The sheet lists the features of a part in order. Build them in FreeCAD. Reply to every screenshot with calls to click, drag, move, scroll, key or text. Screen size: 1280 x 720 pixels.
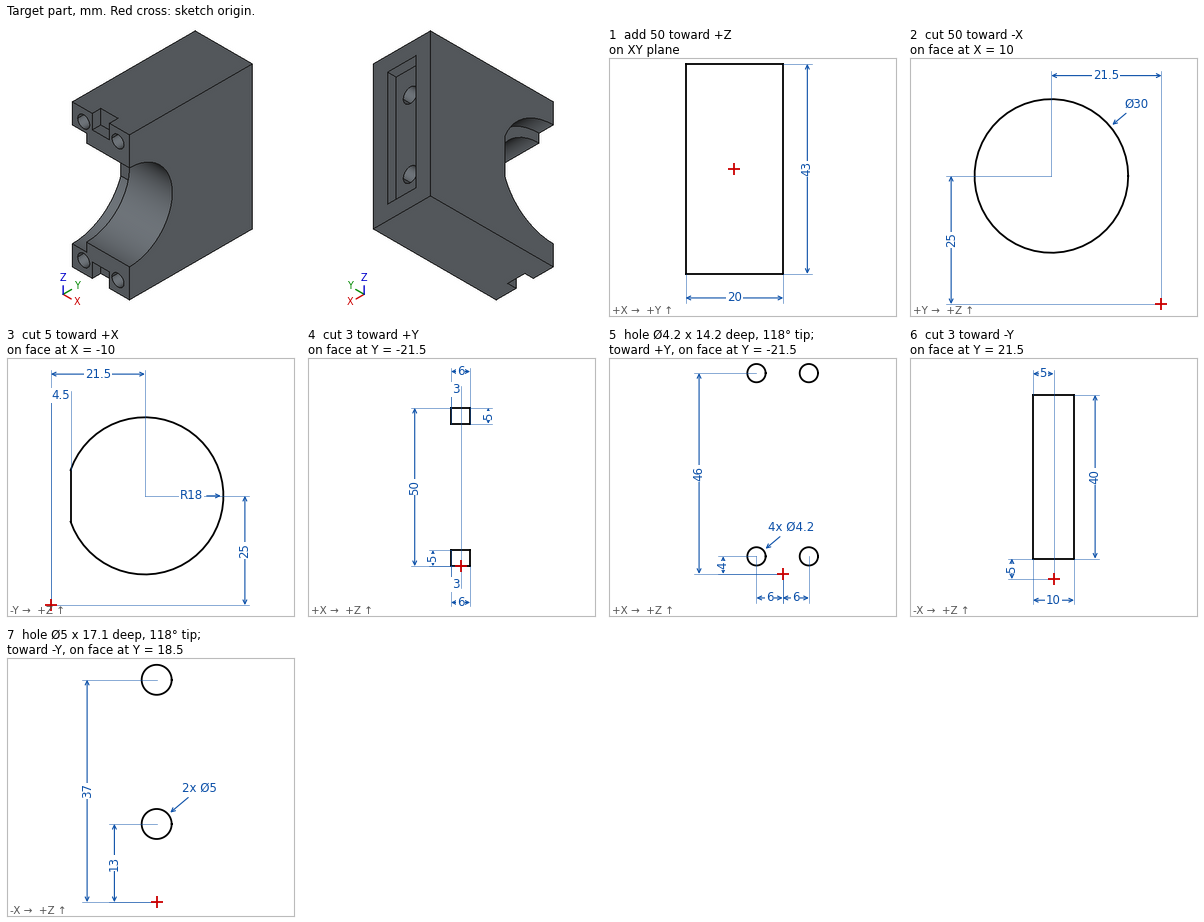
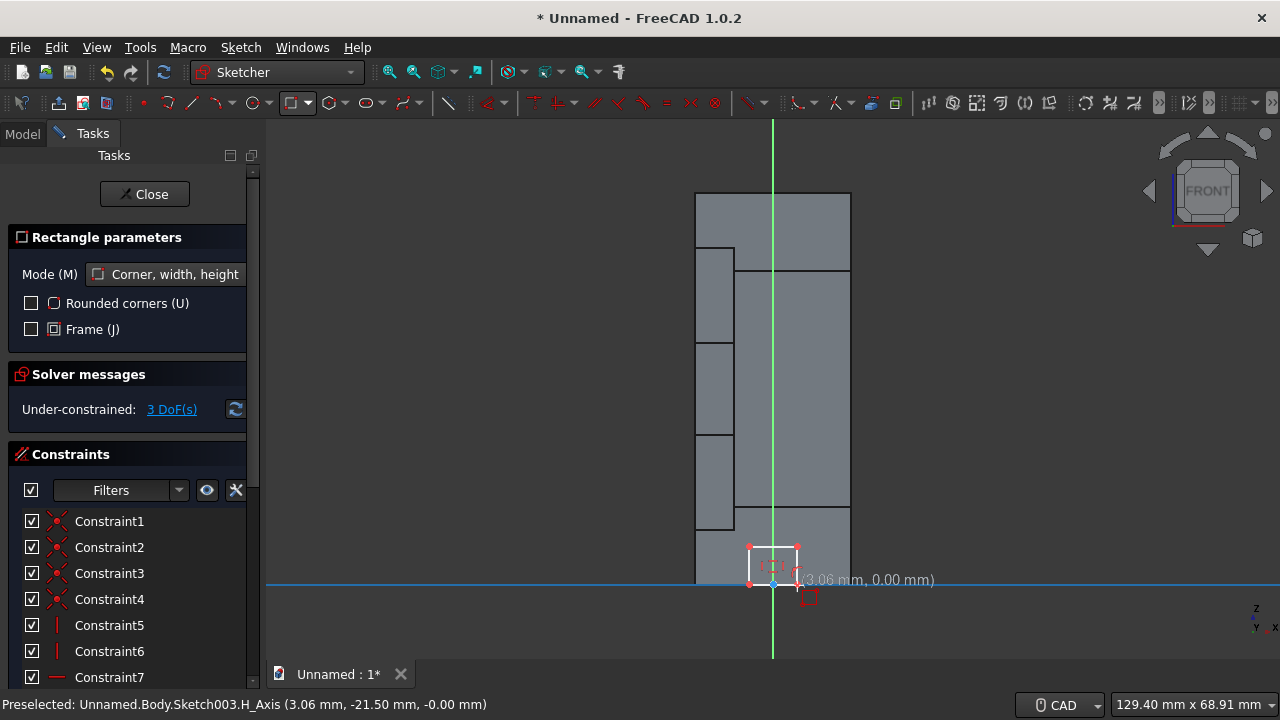
click(749, 193)
move(797, 232)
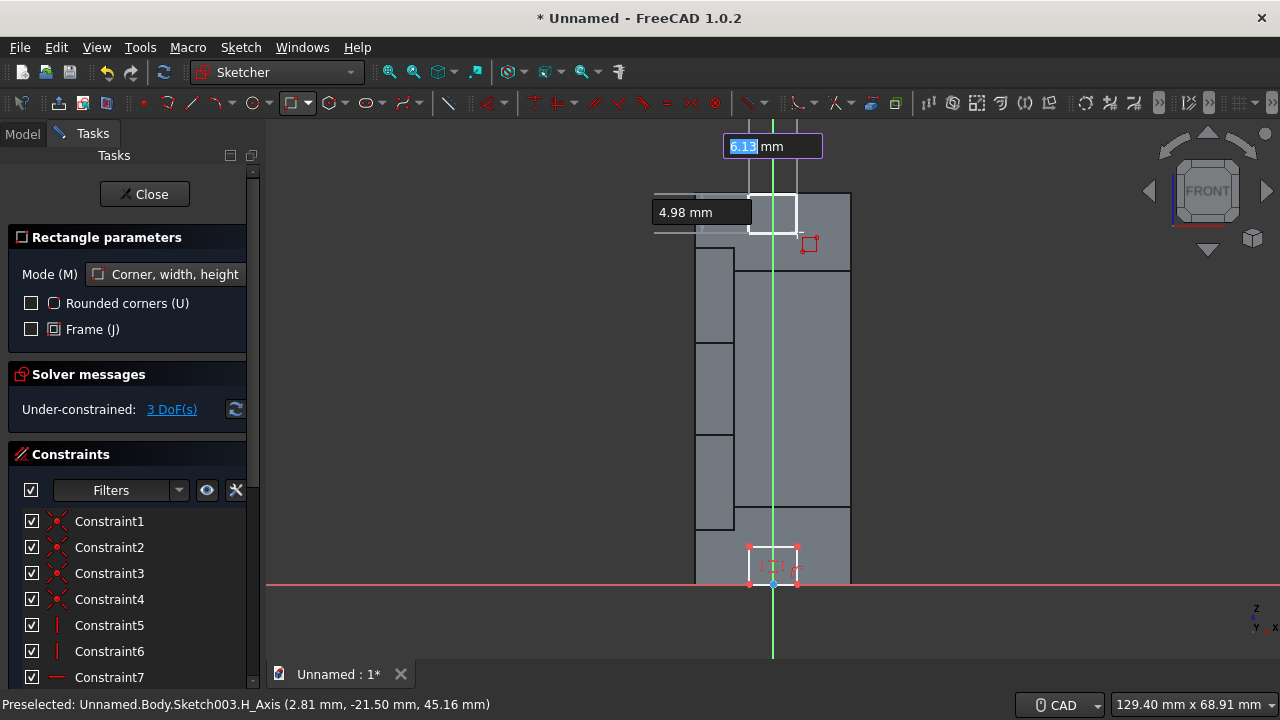
text(6)
key(Tab)
text(5)
key(Return)
key(Escape)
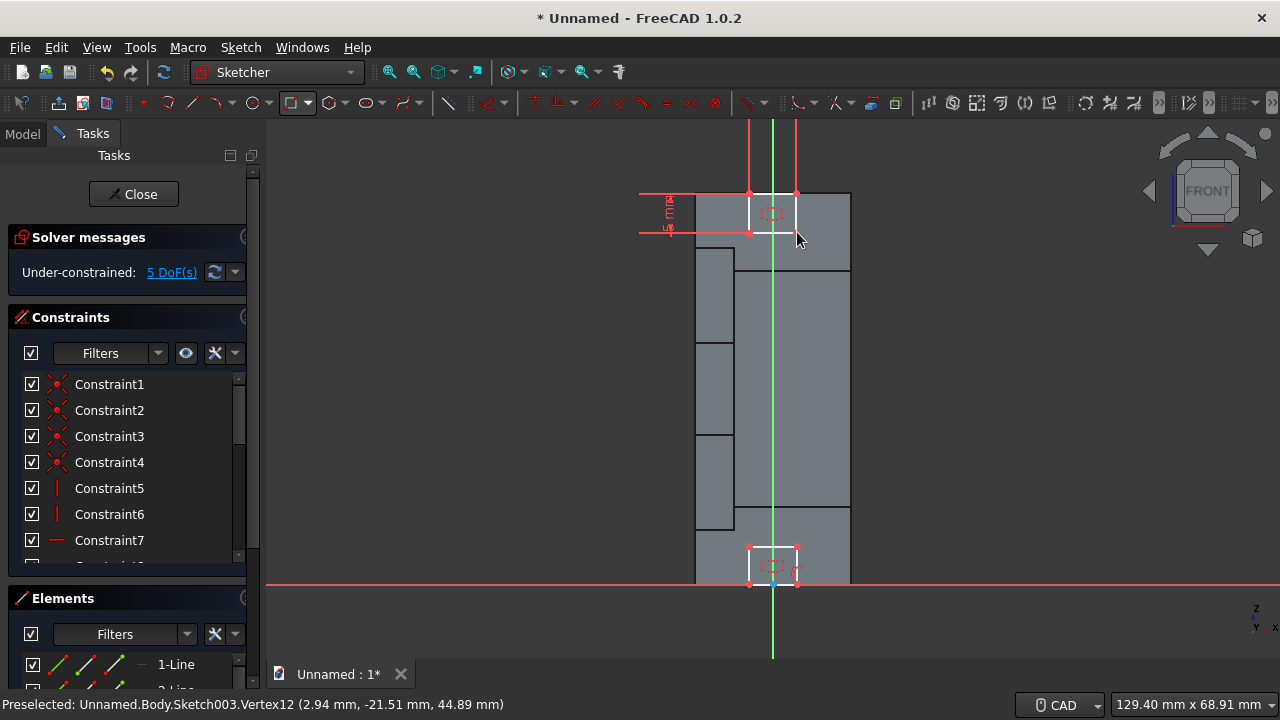
click(488, 104)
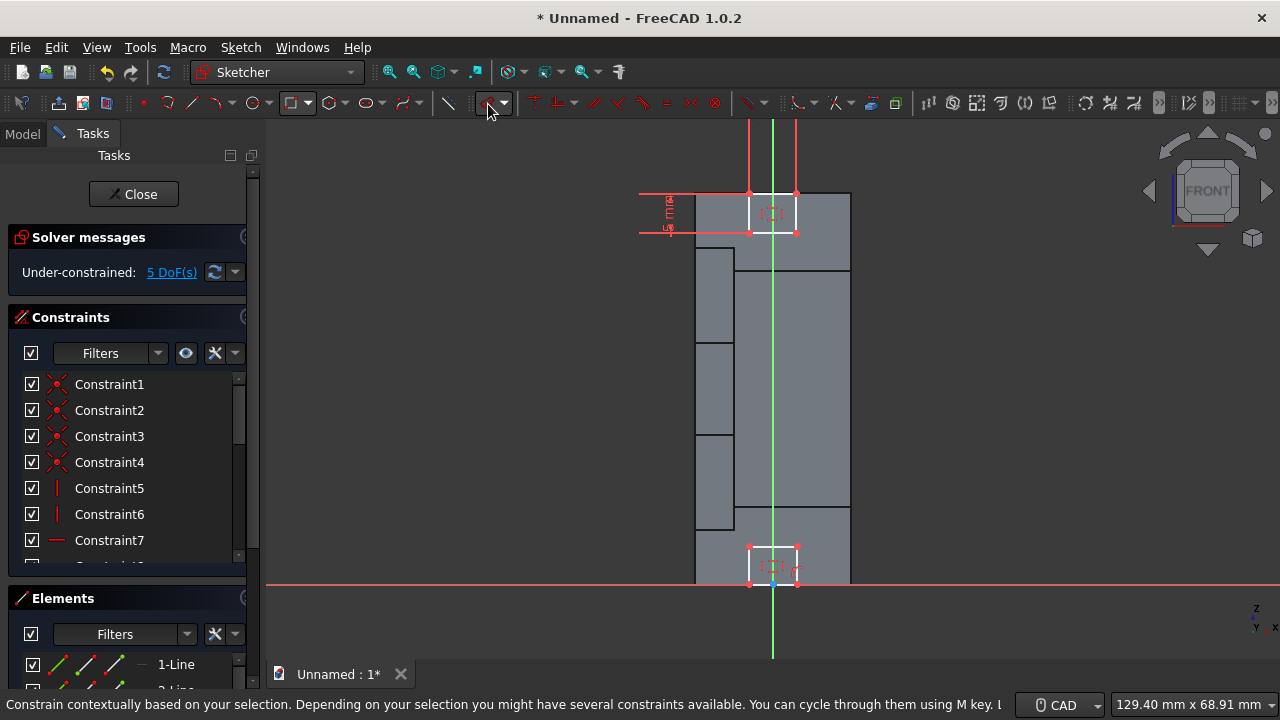
click(749, 558)
click(715, 566)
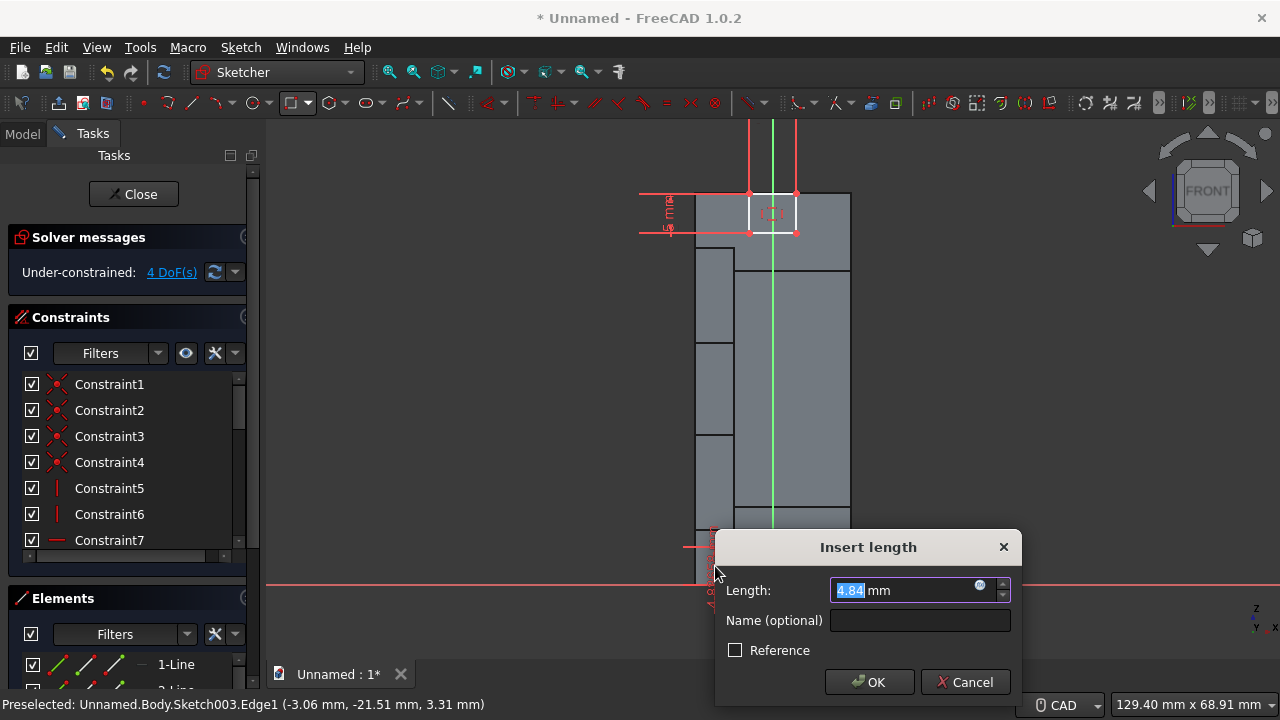
text(5)
key(Return)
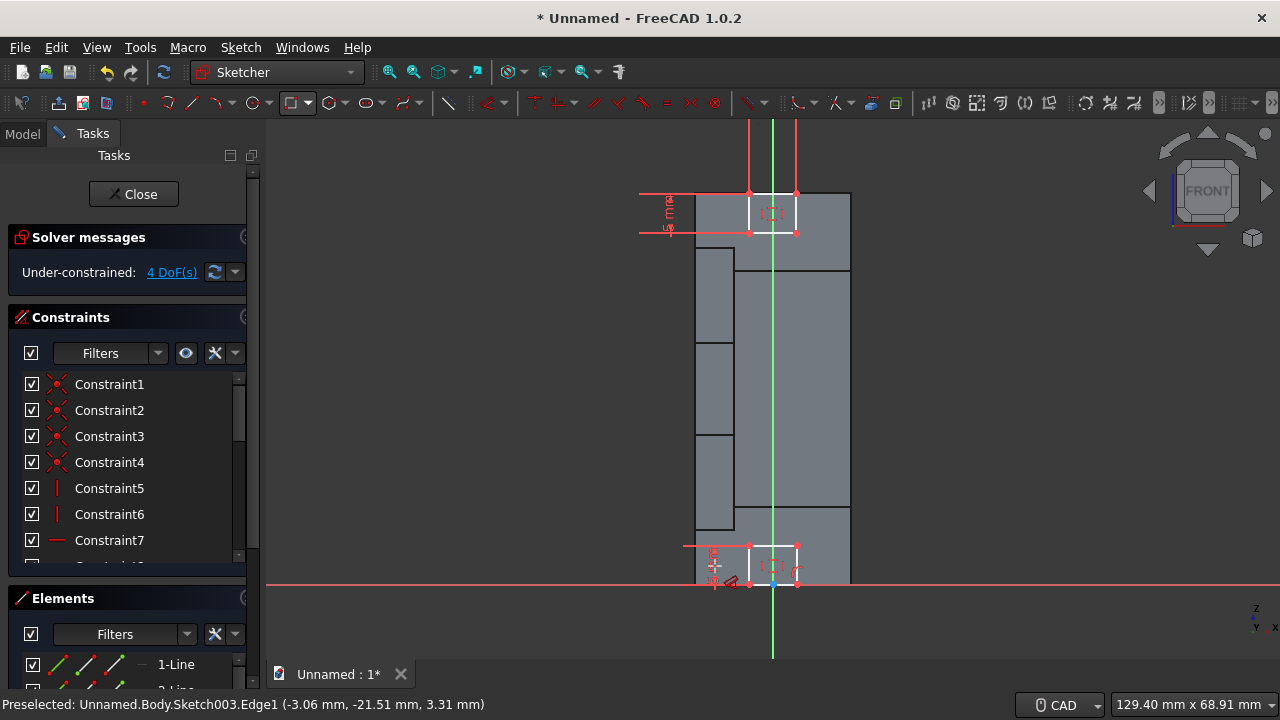
scroll(763, 585, up, 2)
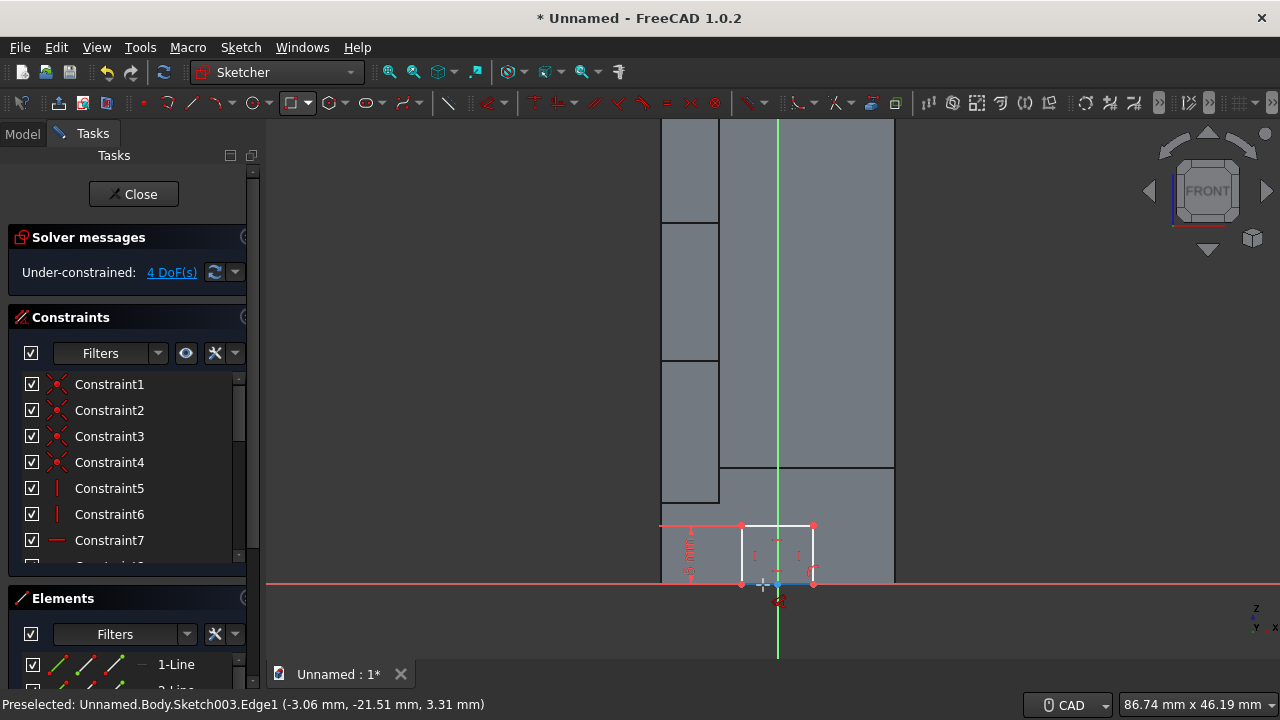
click(763, 584)
click(761, 618)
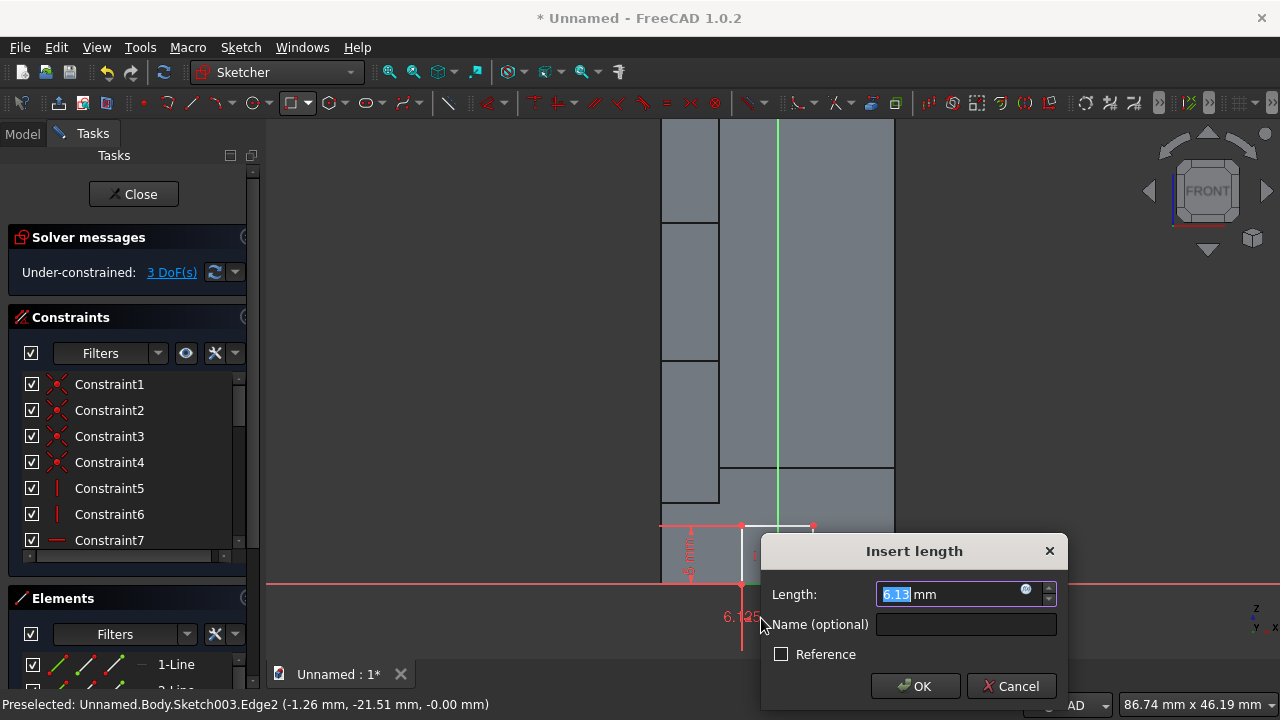
text(6)
key(Return)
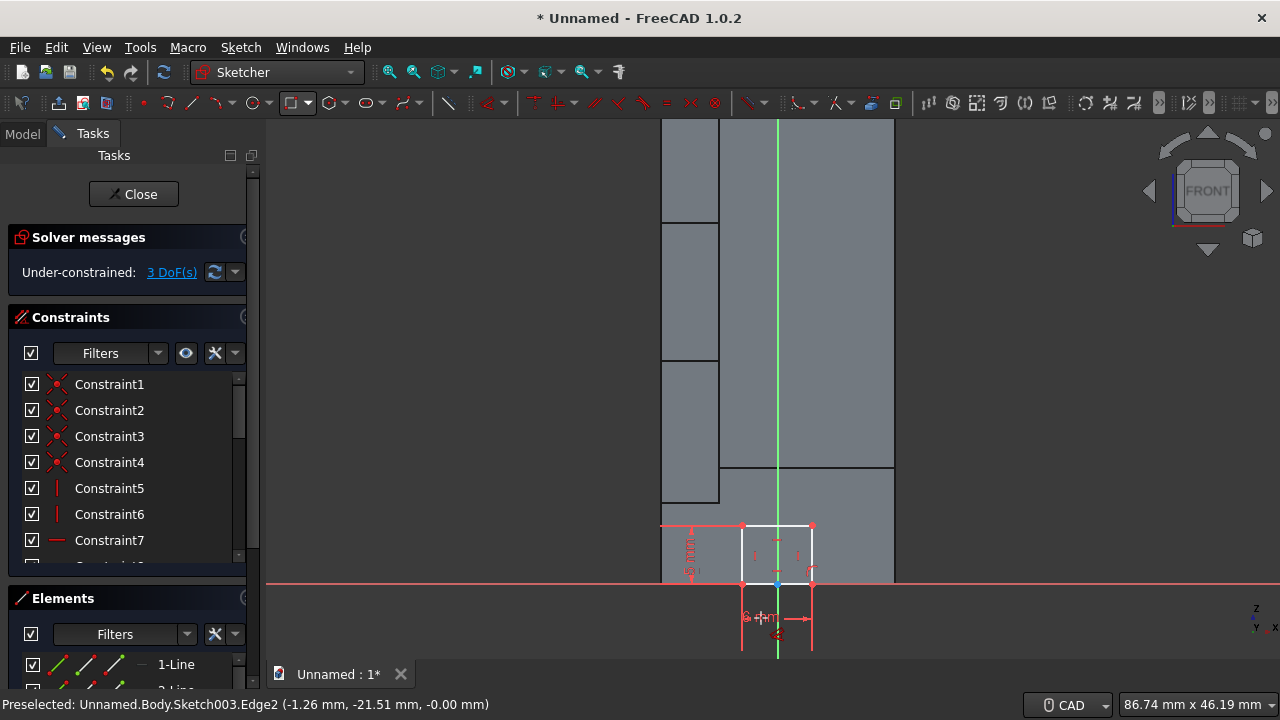
click(742, 526)
click(760, 492)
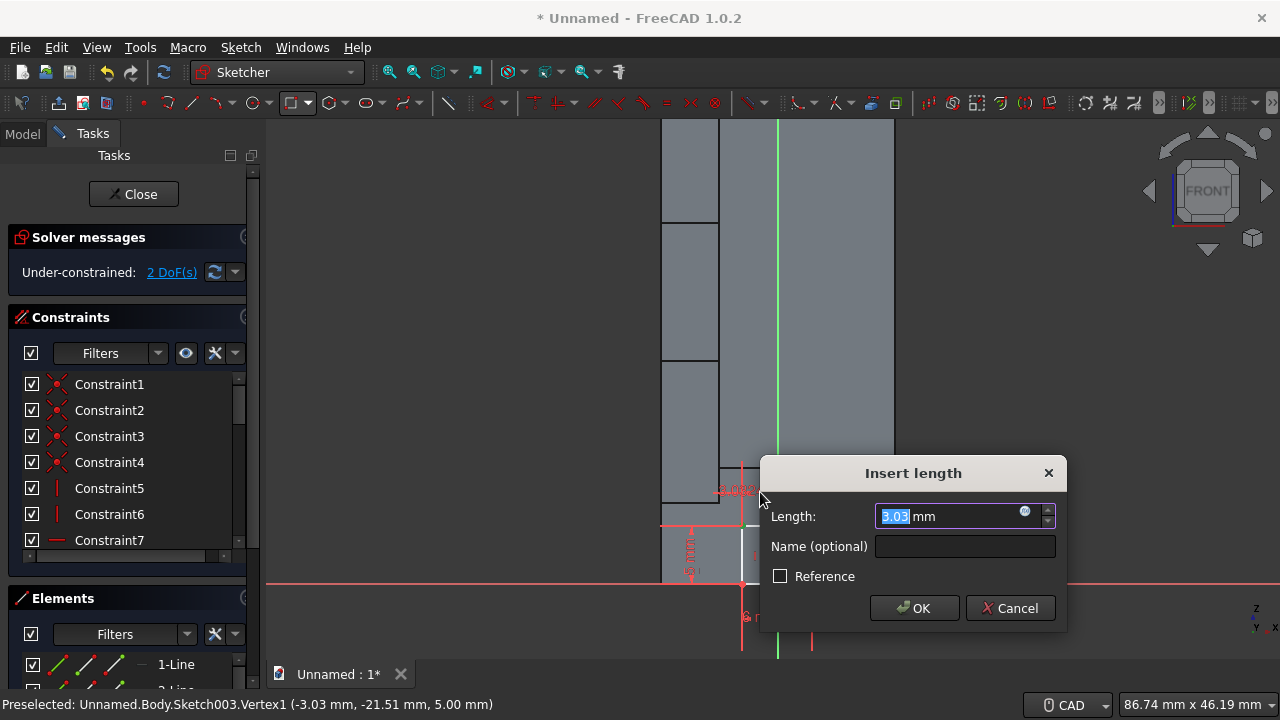
text(3)
key(Return)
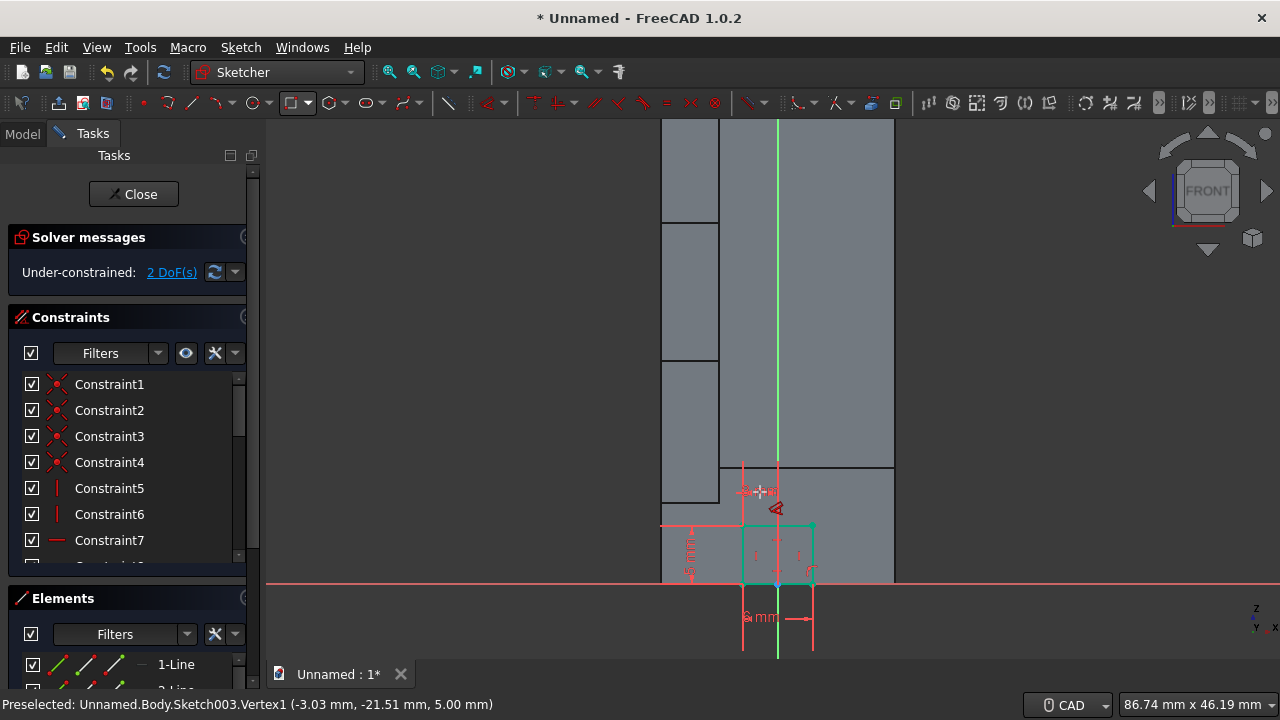
scroll(615, 507, down, 3)